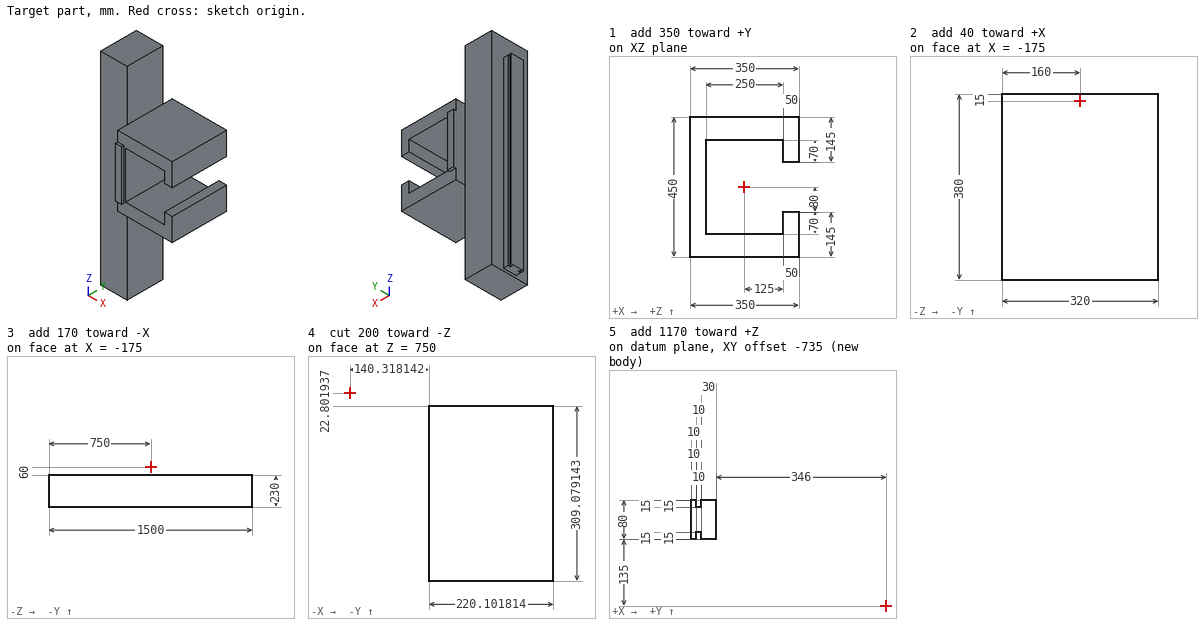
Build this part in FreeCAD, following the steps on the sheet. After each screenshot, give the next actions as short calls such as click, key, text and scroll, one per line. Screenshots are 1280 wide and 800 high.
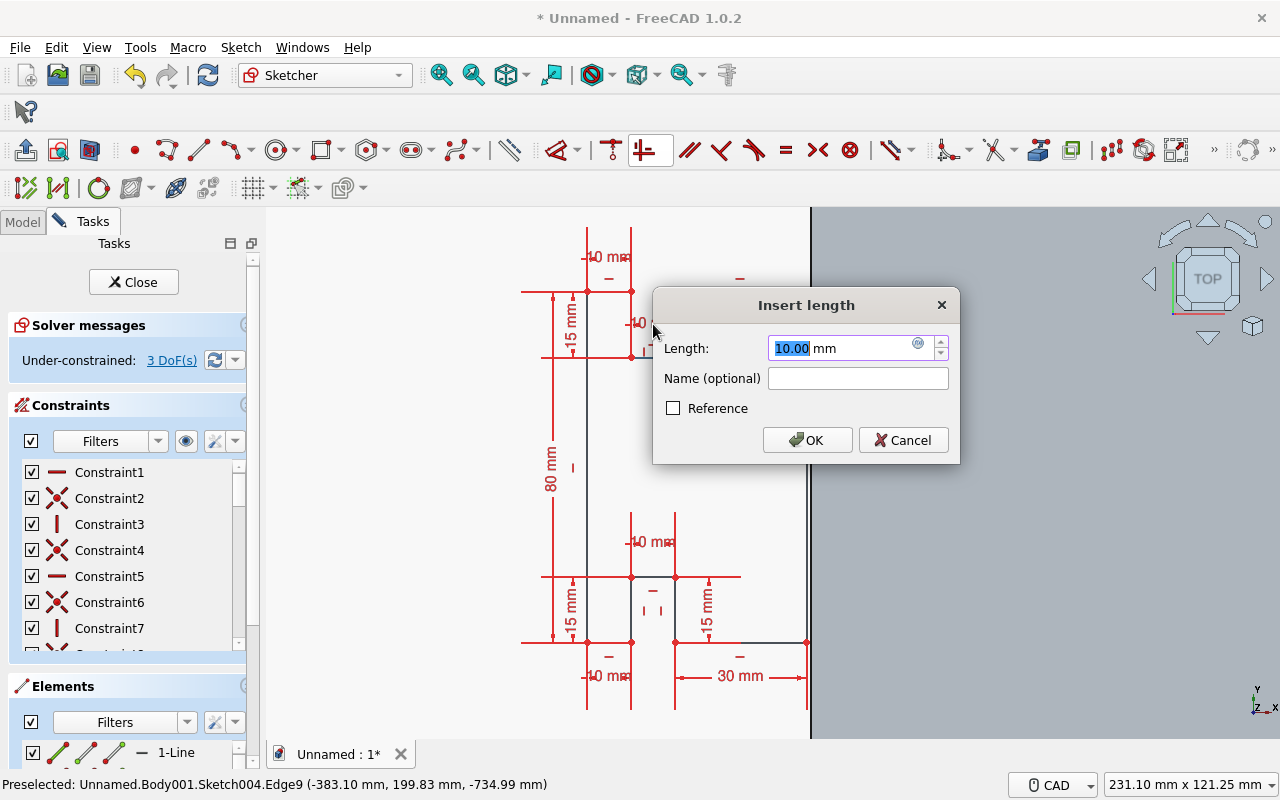
text(10)
key(Return)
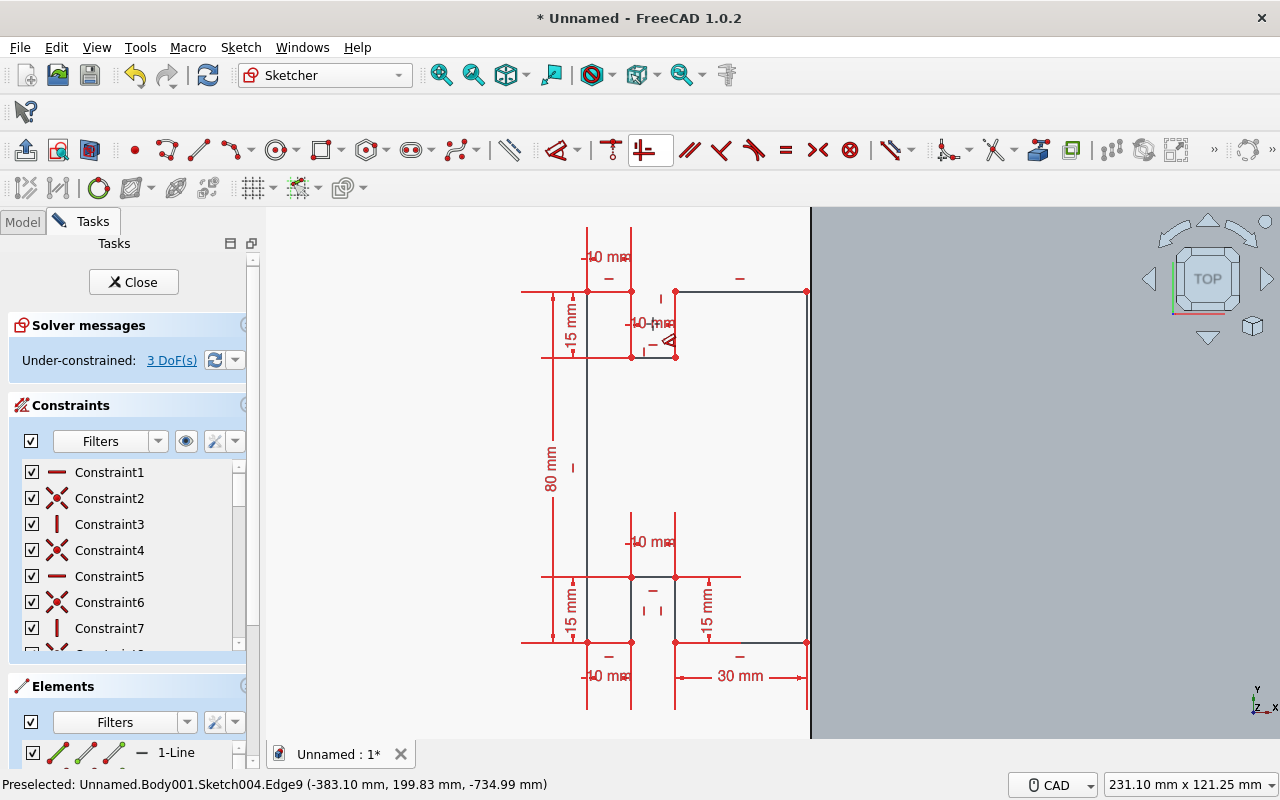
click(675, 338)
click(709, 348)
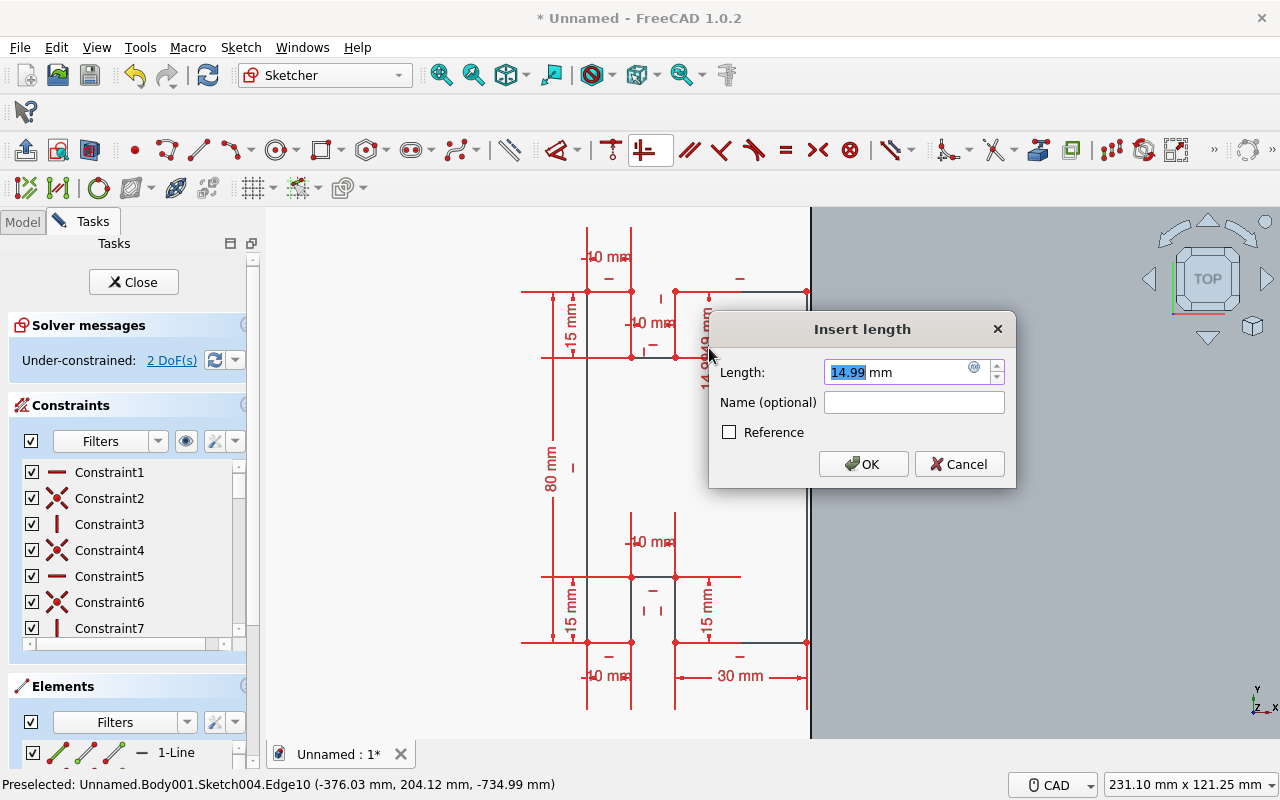
text(15)
key(Return)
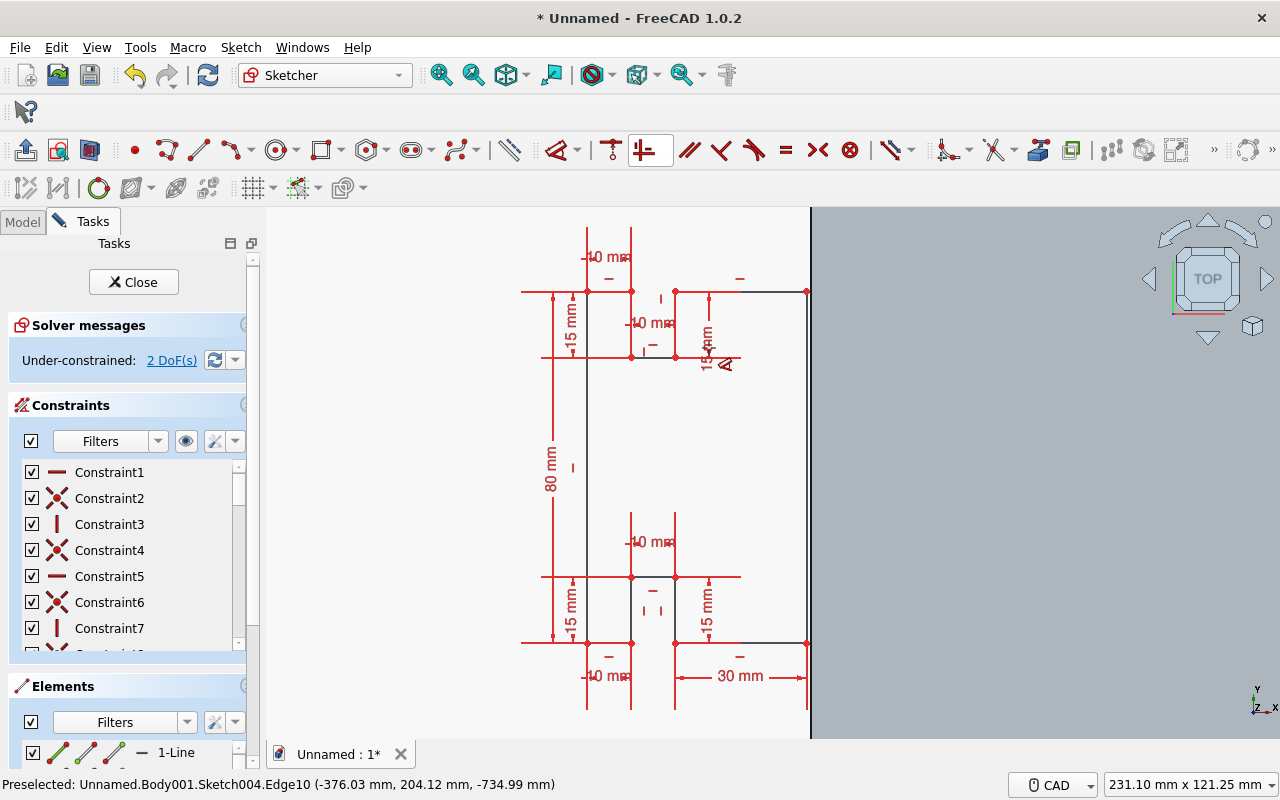
click(807, 643)
click(961, 609)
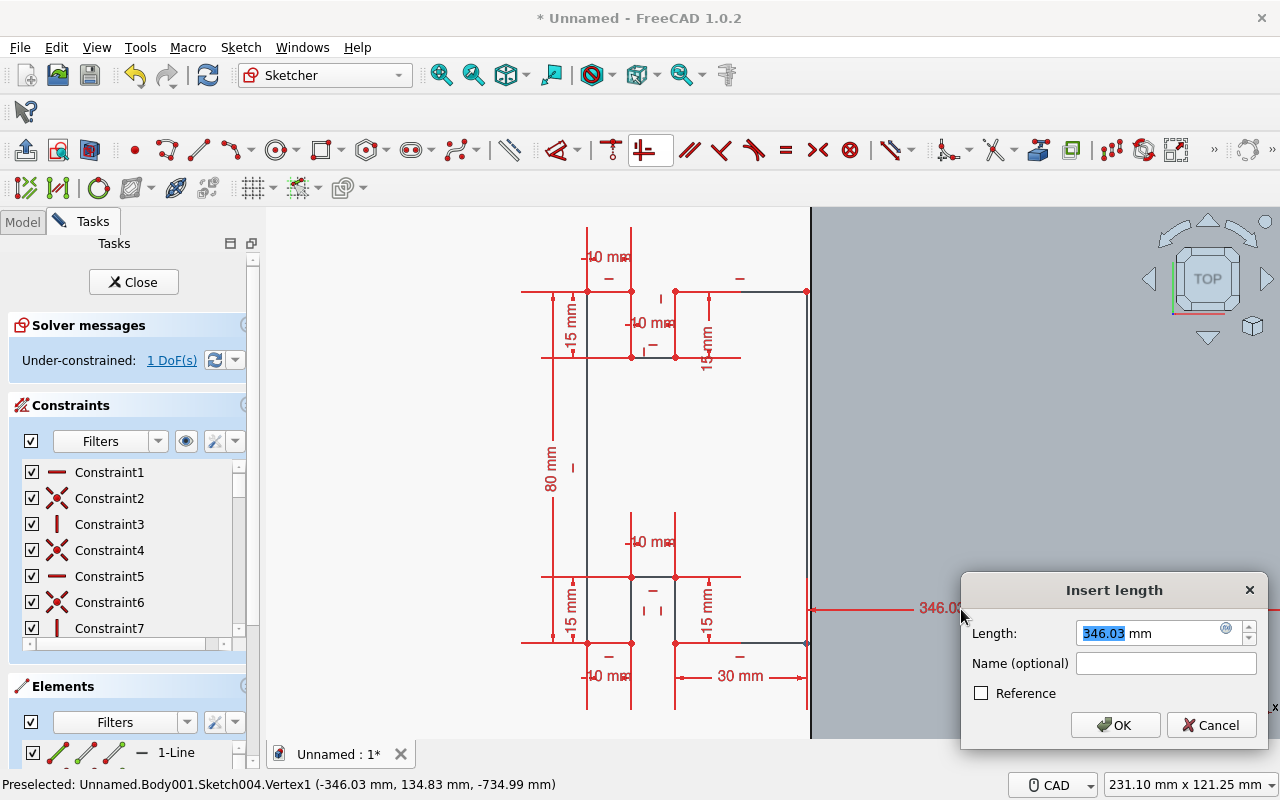
text(346)
key(Return)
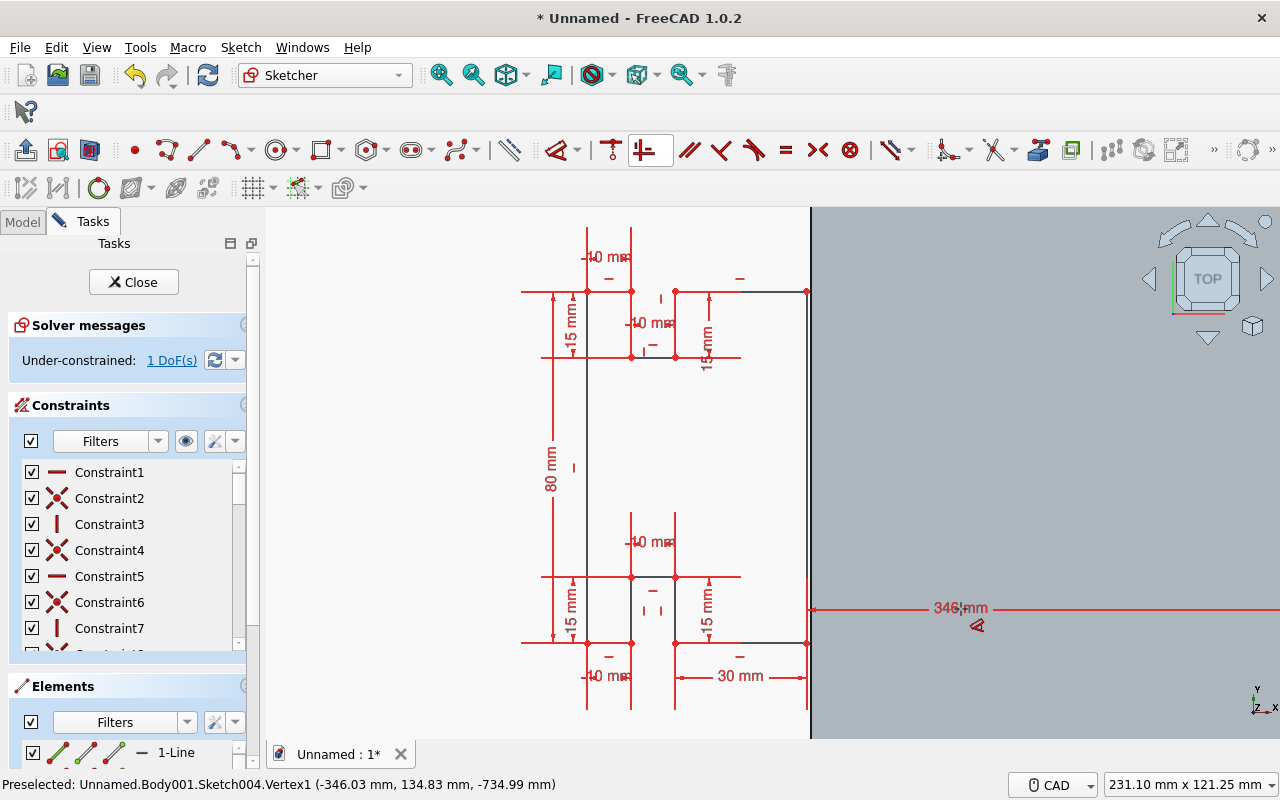
click(807, 643)
click(773, 701)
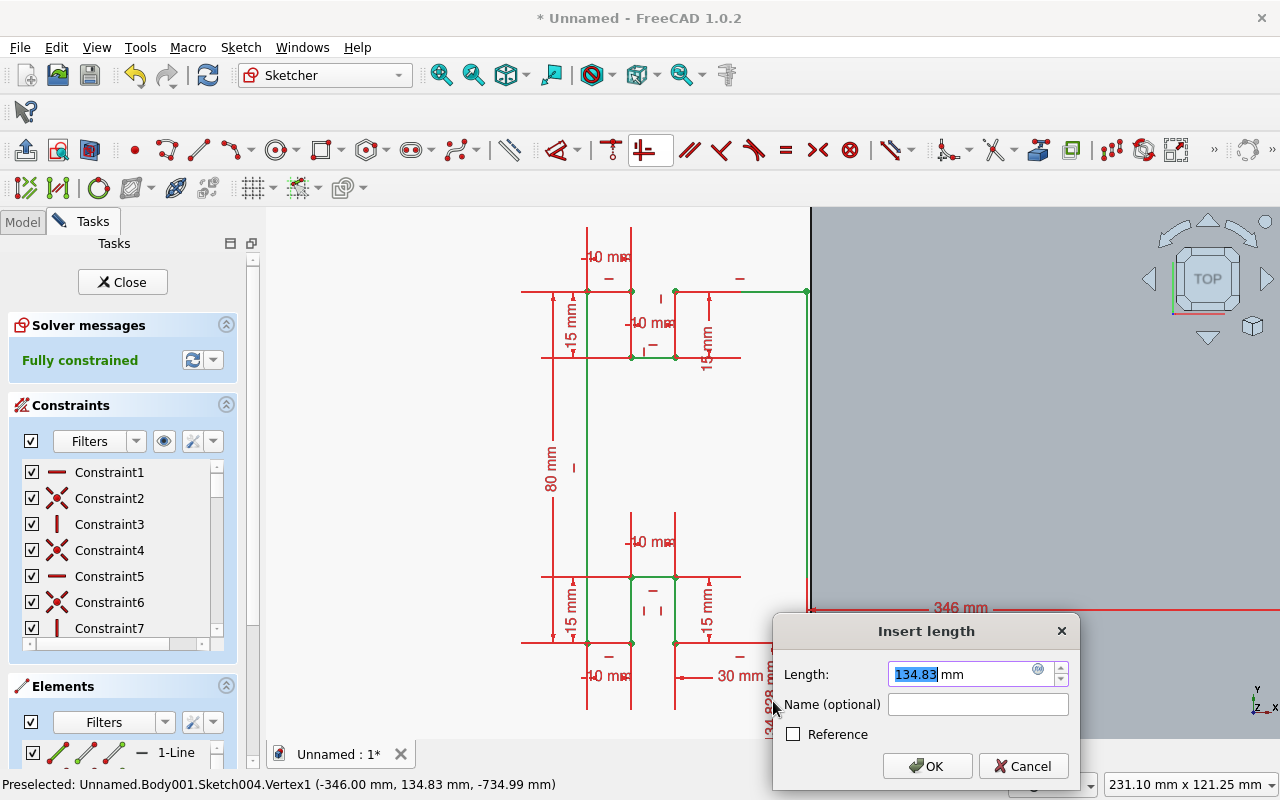
text(135)
key(Return)
key(Escape)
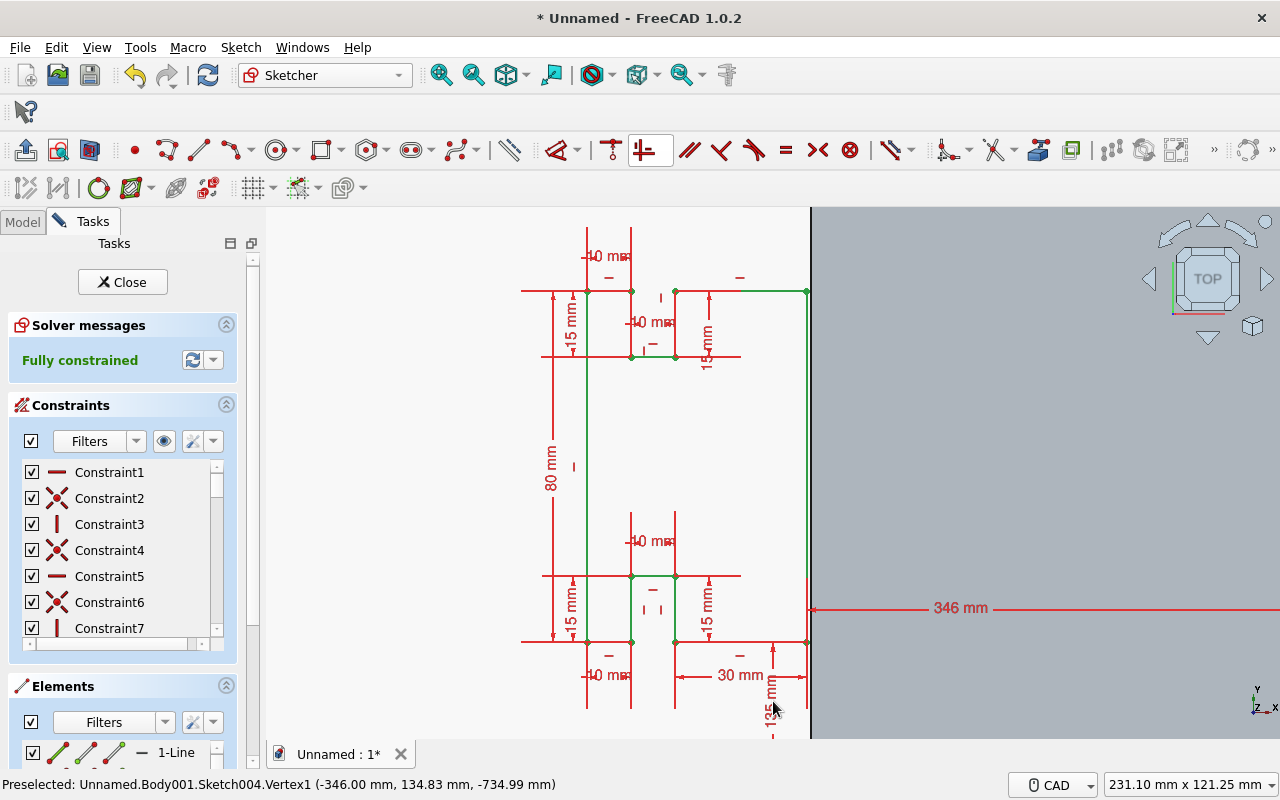
click(123, 282)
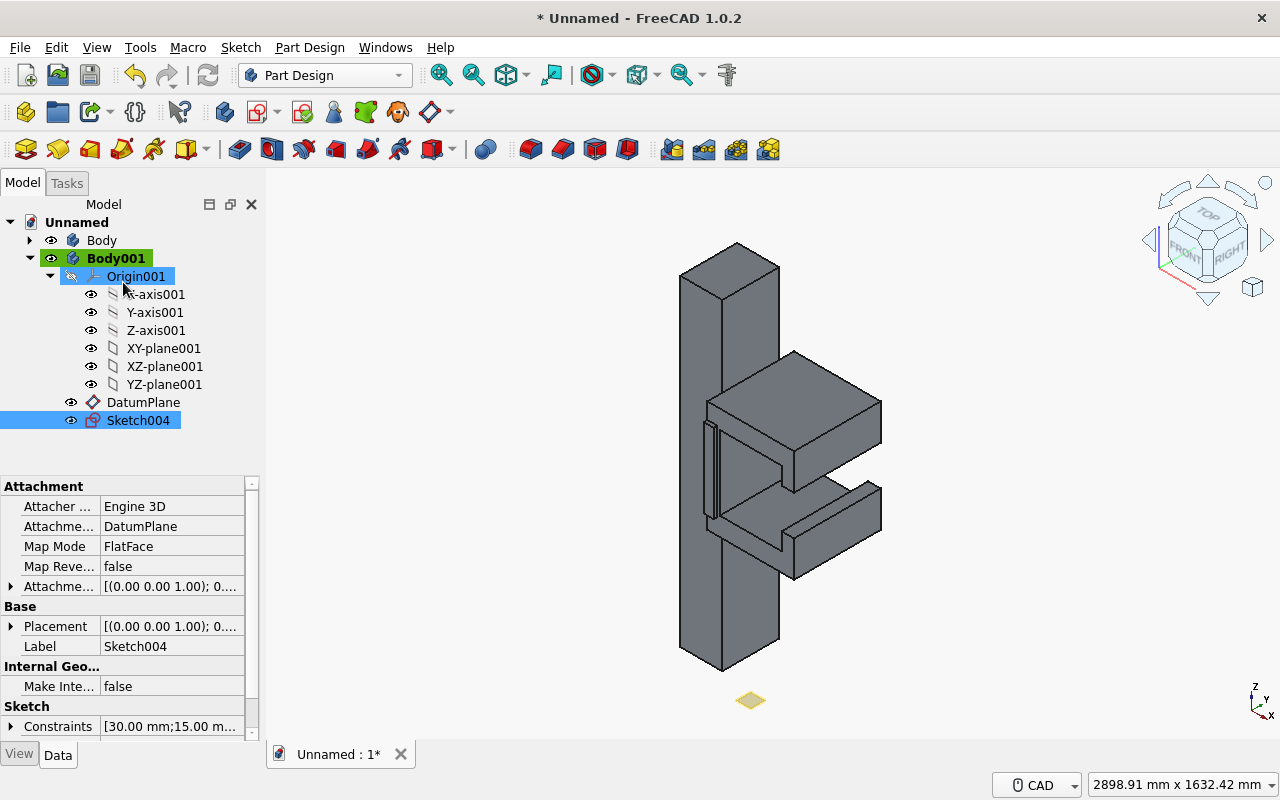
click(26, 150)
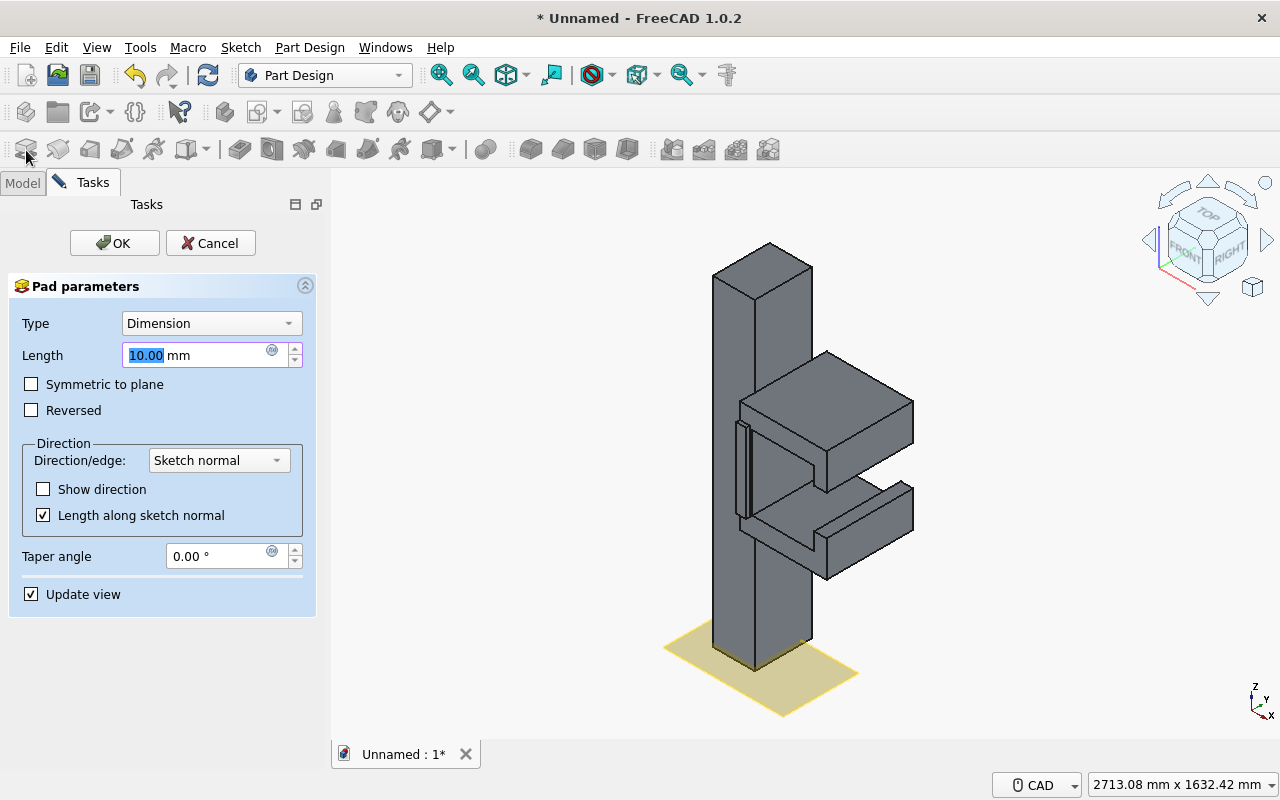
text(1170)
key(Tab)